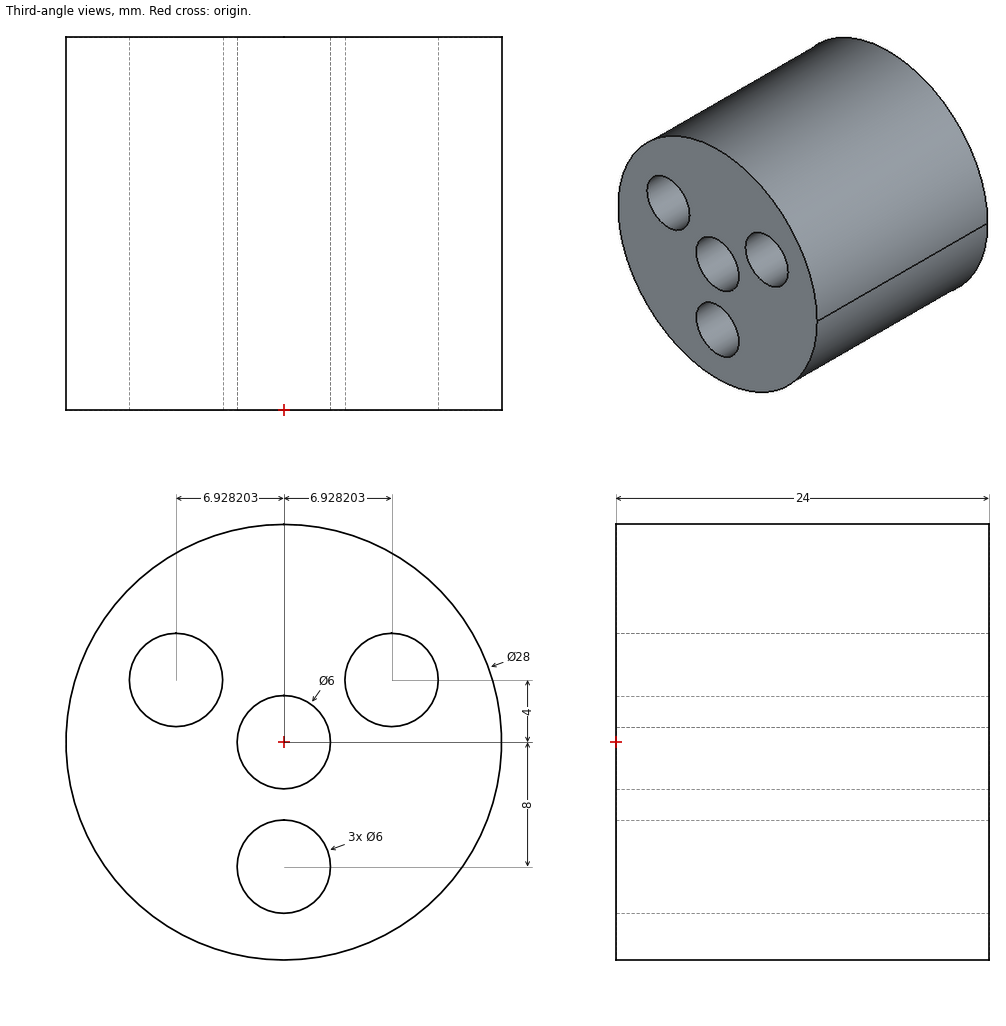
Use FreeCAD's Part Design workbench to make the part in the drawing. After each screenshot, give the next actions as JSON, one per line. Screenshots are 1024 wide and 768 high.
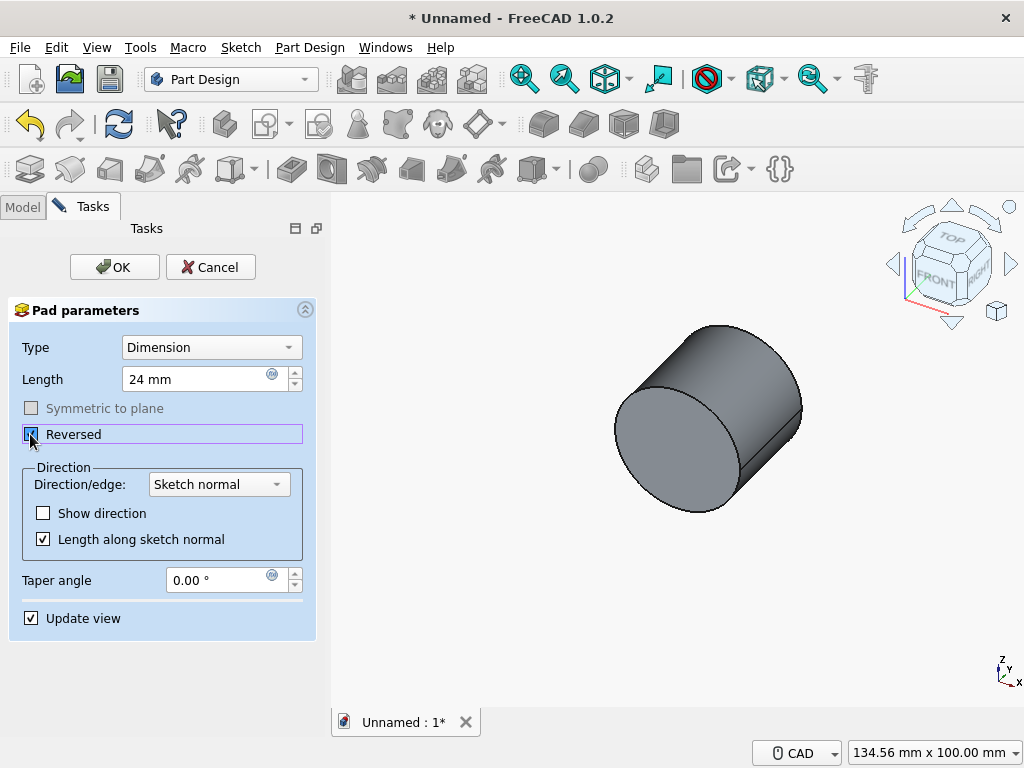
{"action": "left_click", "coordinate": [115, 267]}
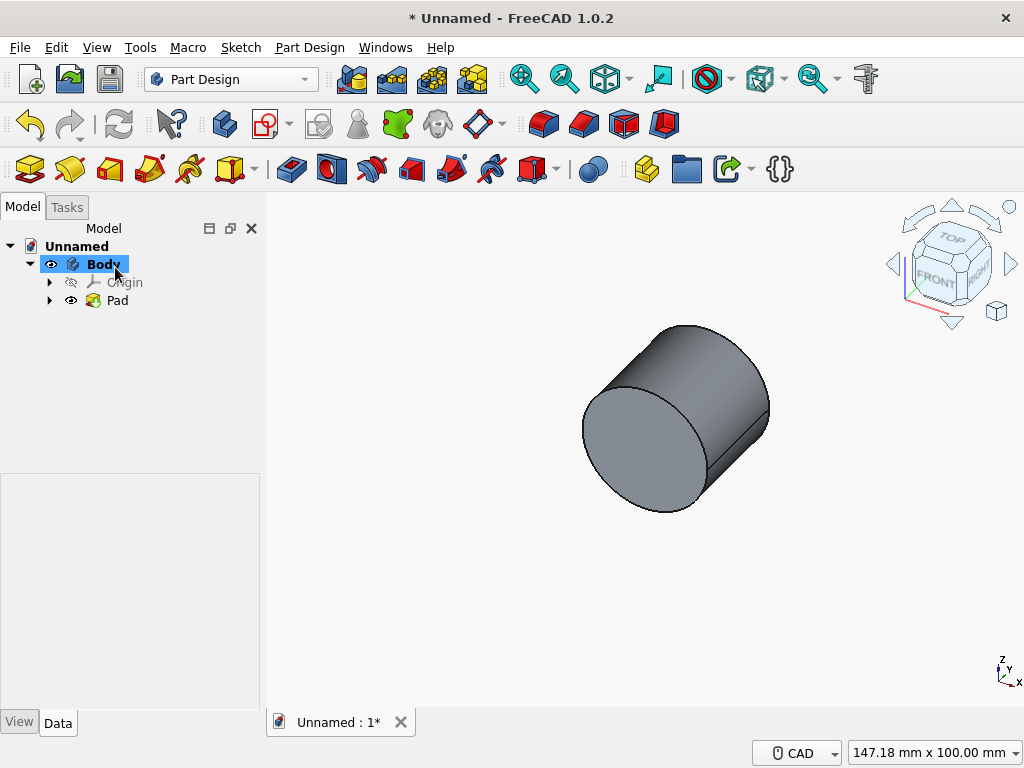
{"action": "left_click", "coordinate": [526, 80]}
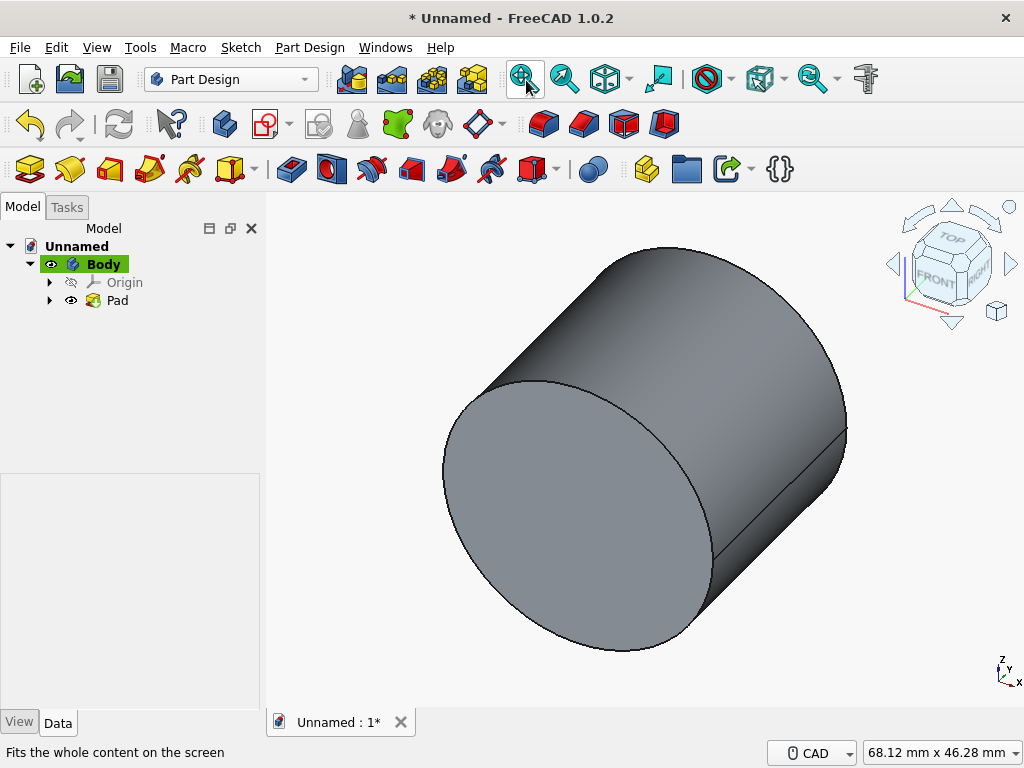
{"action": "key", "text": "4"}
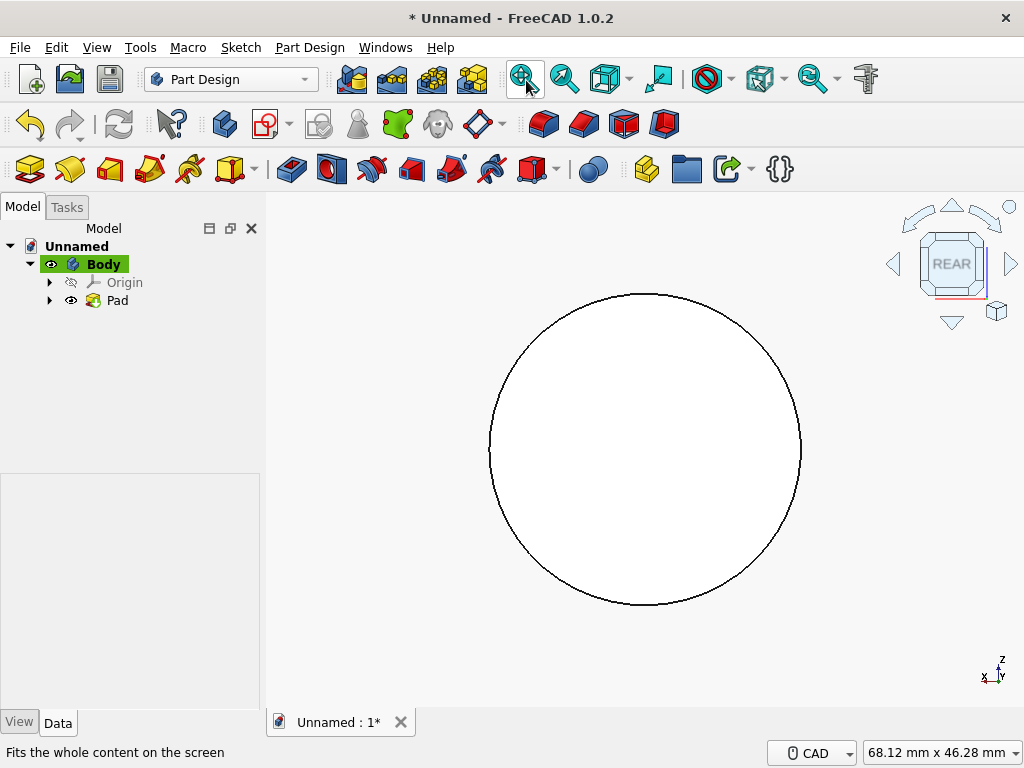
{"action": "left_click", "coordinate": [645, 449]}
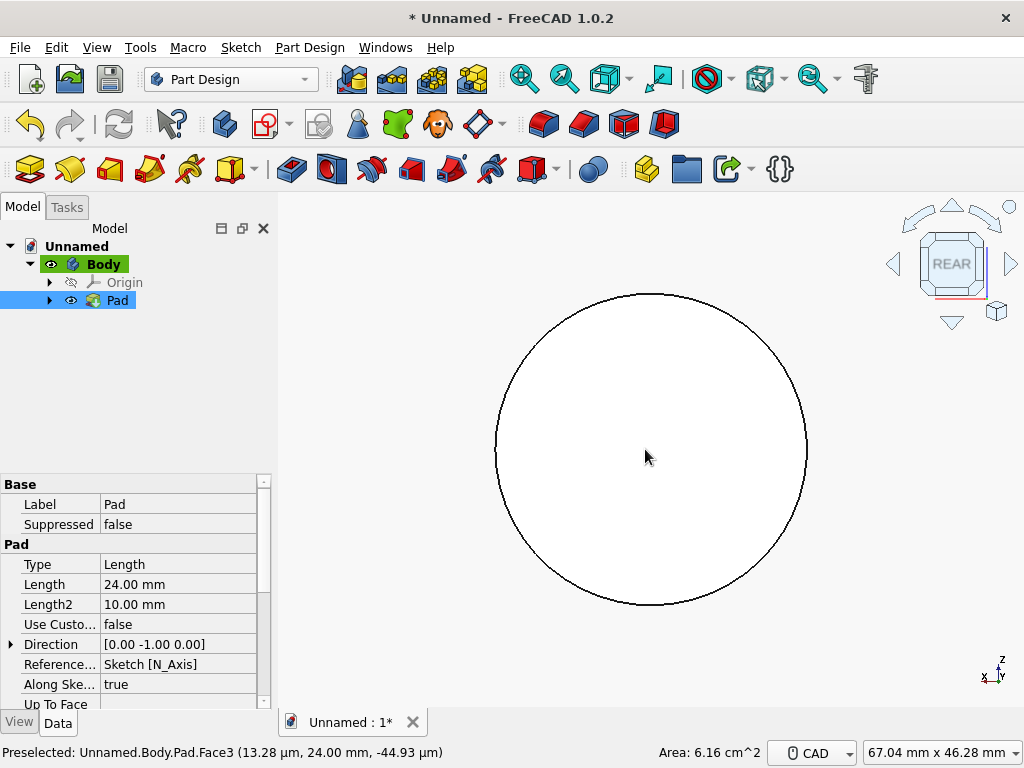
{"action": "left_click", "coordinate": [266, 124]}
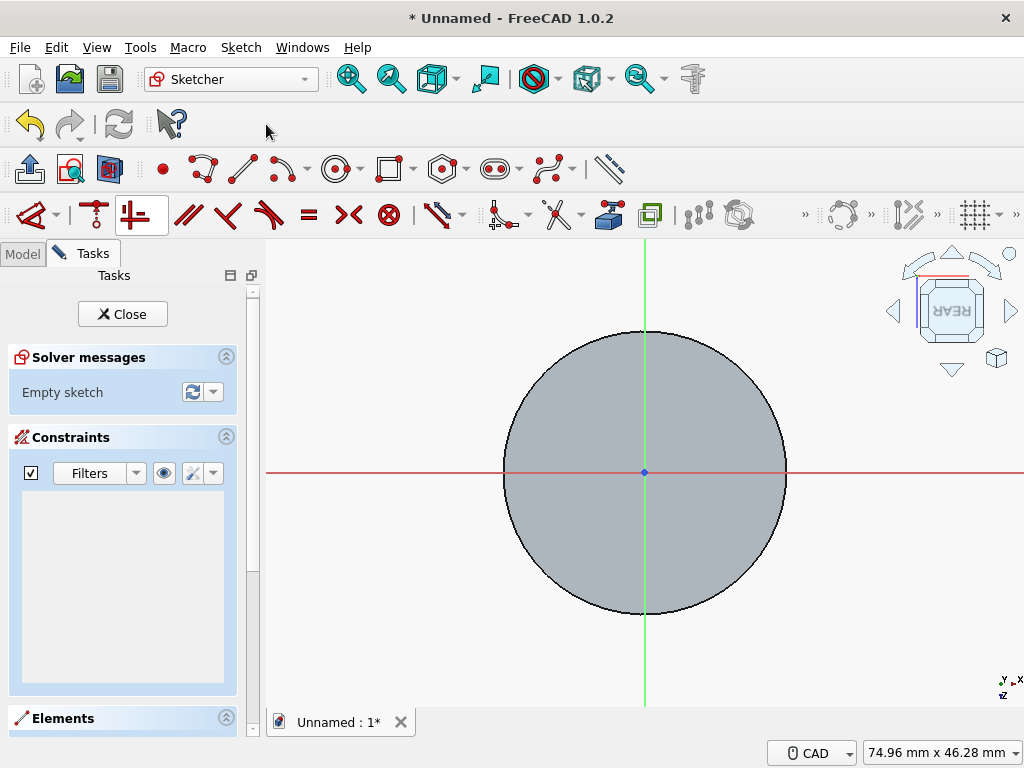
{"action": "scroll", "coordinate": [784, 412], "scroll_direction": "up", "scroll_amount": 2}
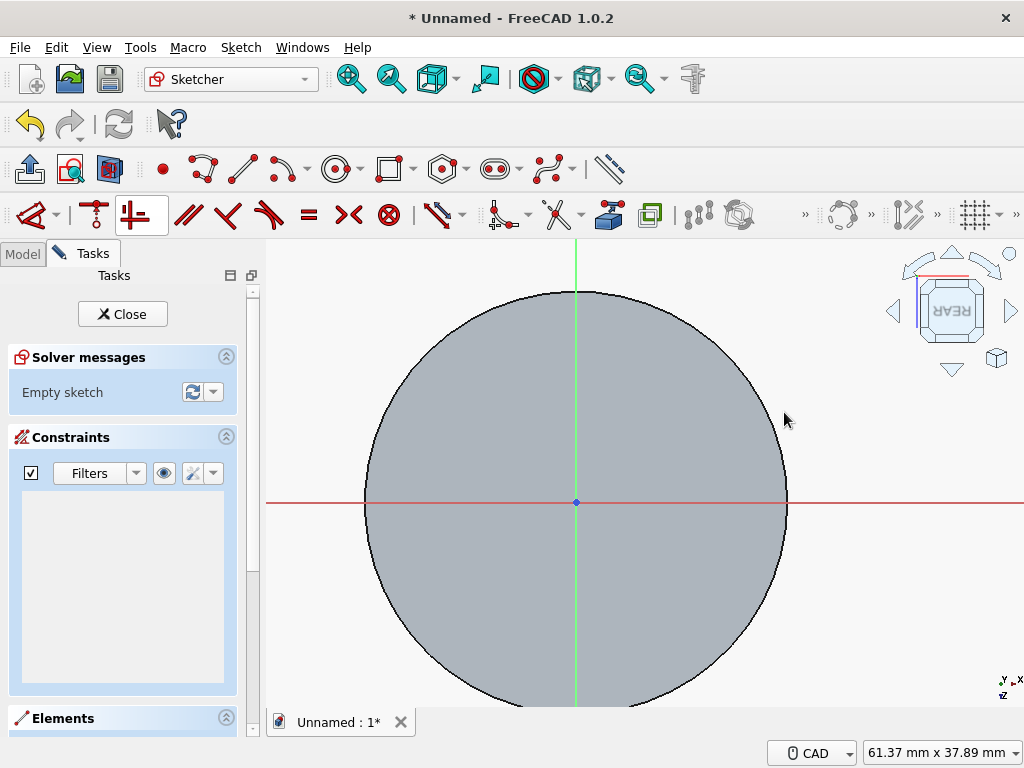
{"action": "key", "text": "g c"}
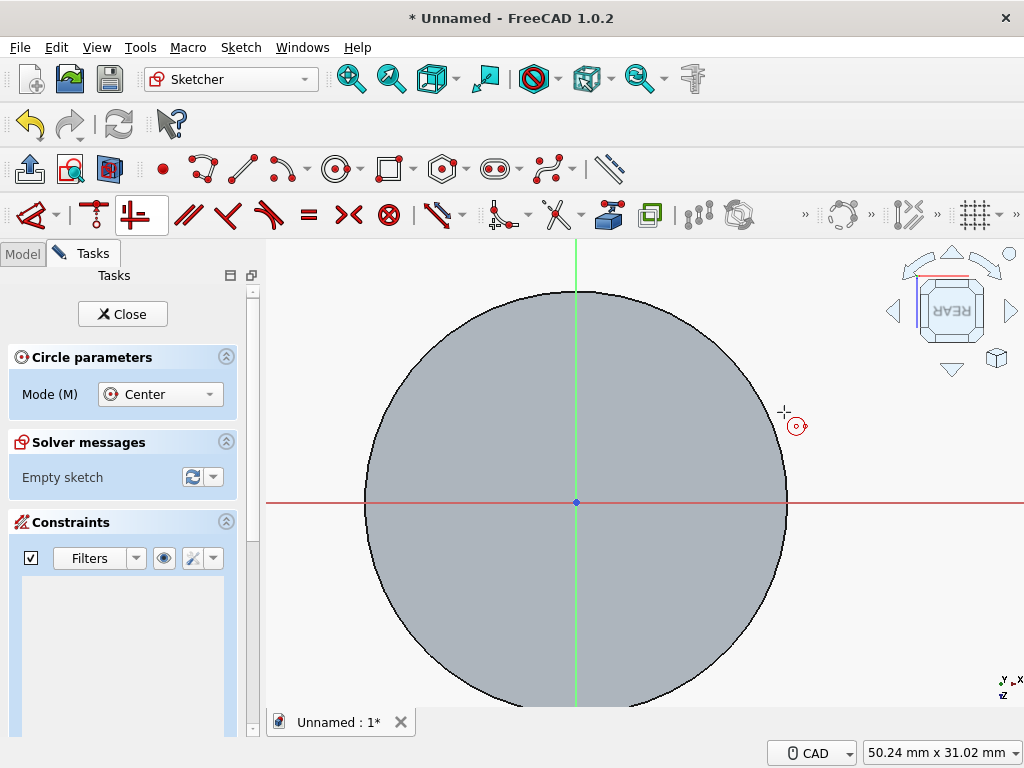
{"action": "left_click", "coordinate": [576, 382]}
{"action": "mouse_move", "coordinate": [608, 350]}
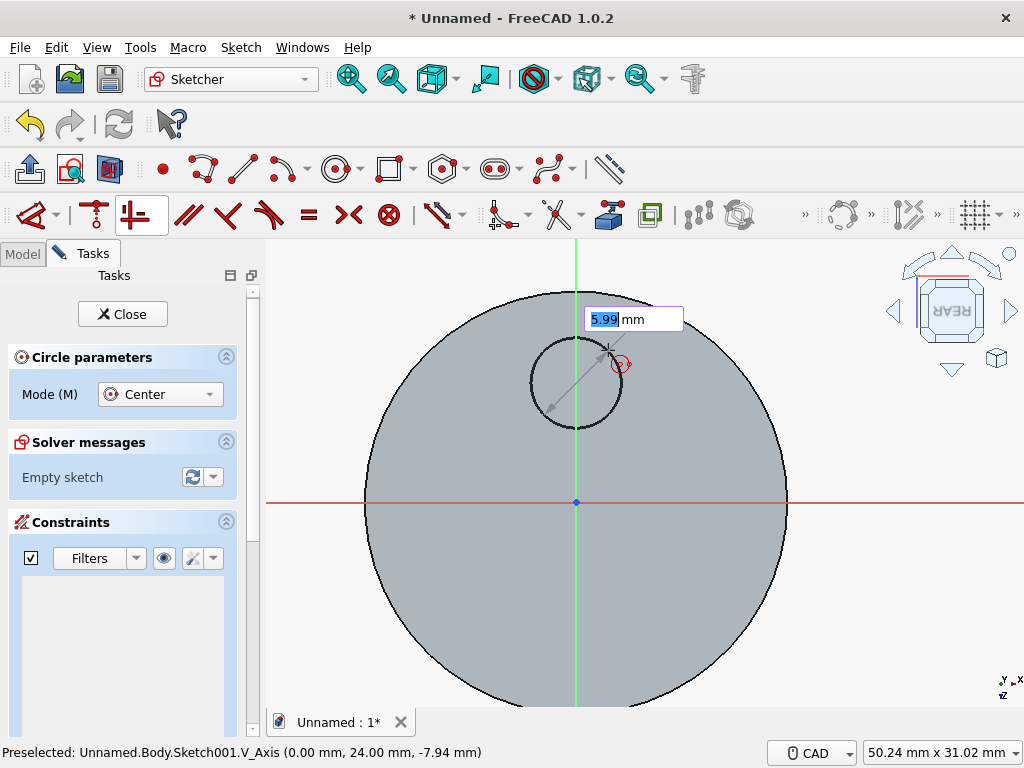
{"action": "type", "text": "6"}
{"action": "key", "text": "Return"}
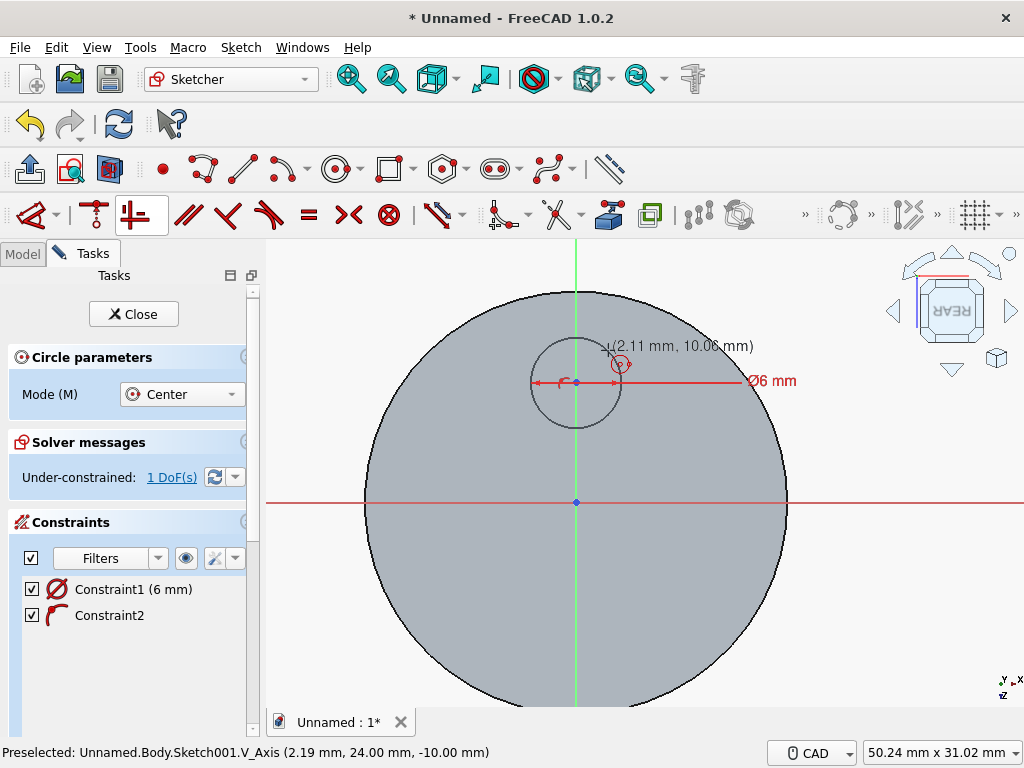
{"action": "left_click", "coordinate": [681, 563]}
{"action": "mouse_move", "coordinate": [713, 531]}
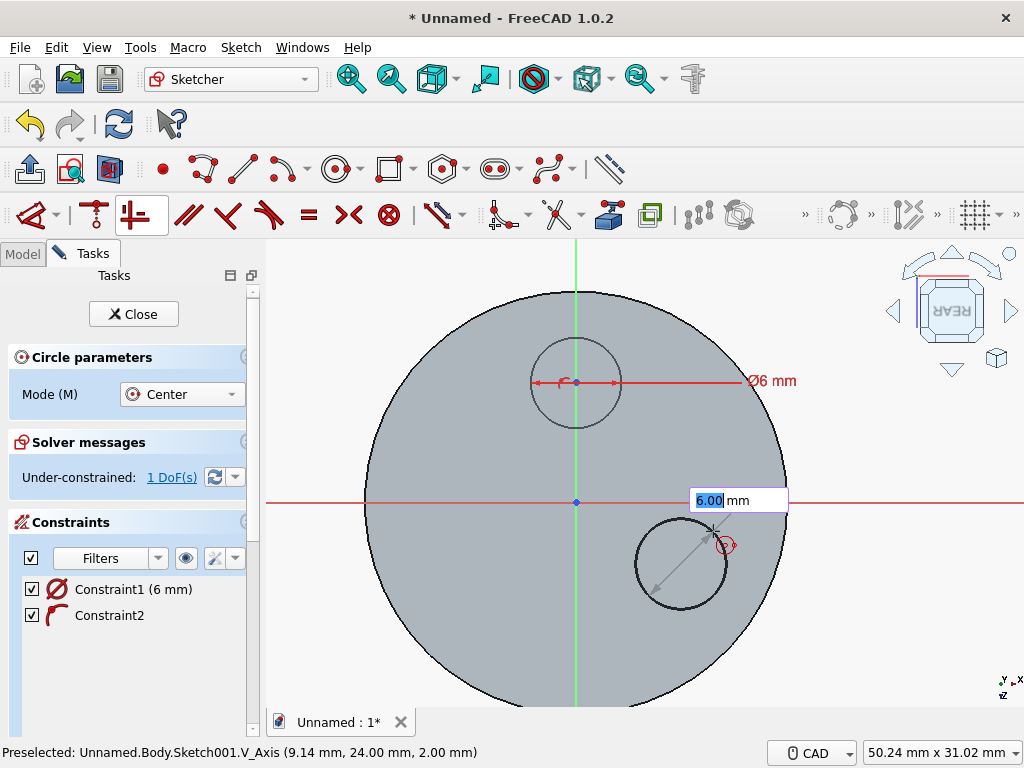
{"action": "type", "text": "6"}
{"action": "key", "text": "Return"}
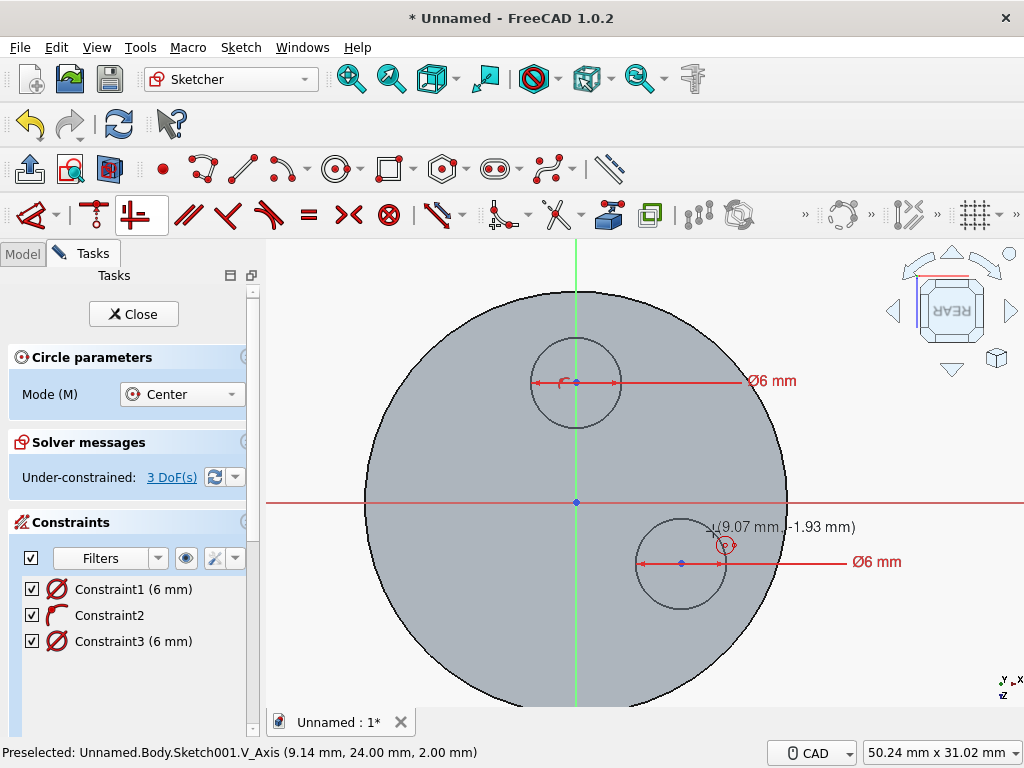
{"action": "left_click", "coordinate": [472, 563]}
{"action": "mouse_move", "coordinate": [504, 531]}